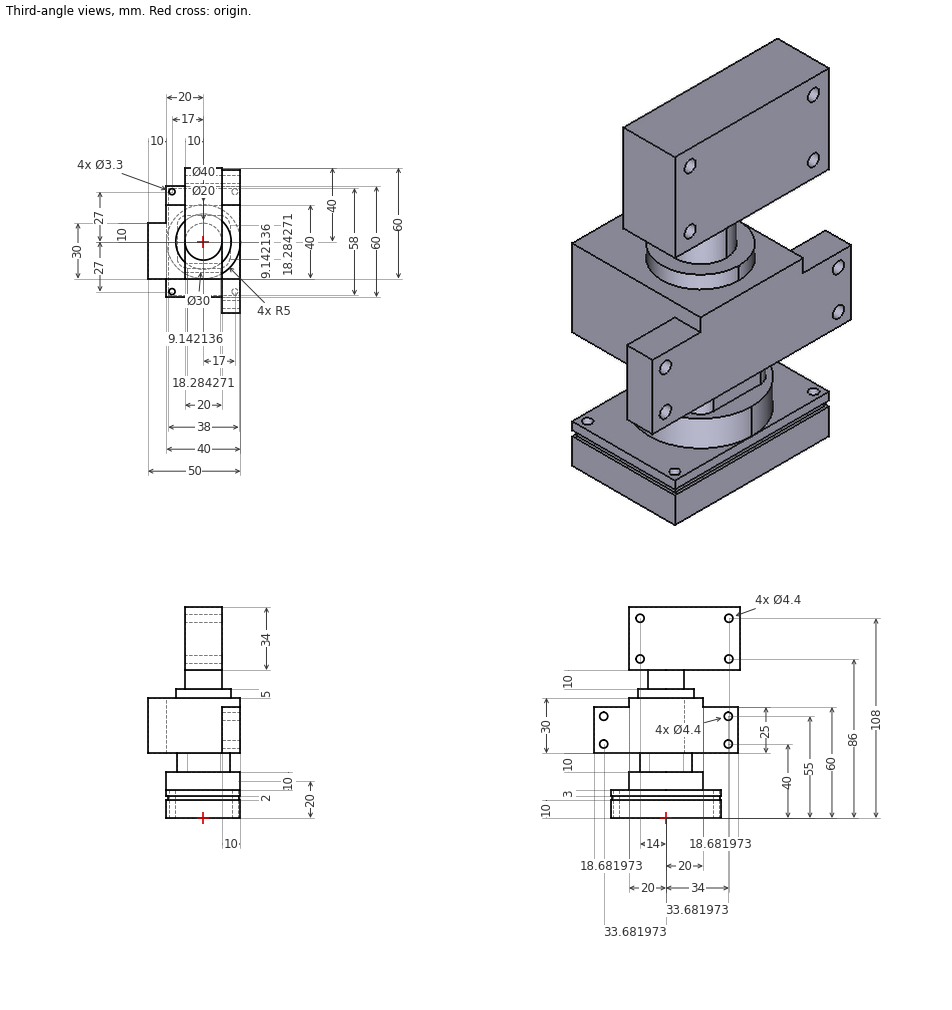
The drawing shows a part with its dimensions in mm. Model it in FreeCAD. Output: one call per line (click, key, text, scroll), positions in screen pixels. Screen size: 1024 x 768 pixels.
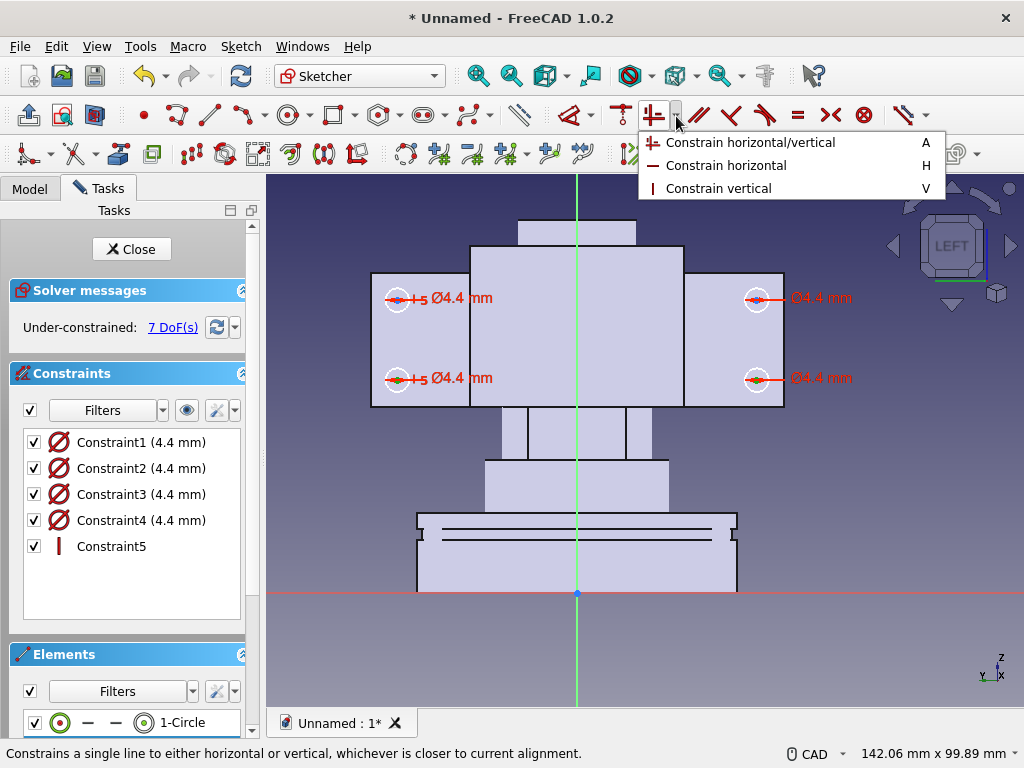
click(792, 166)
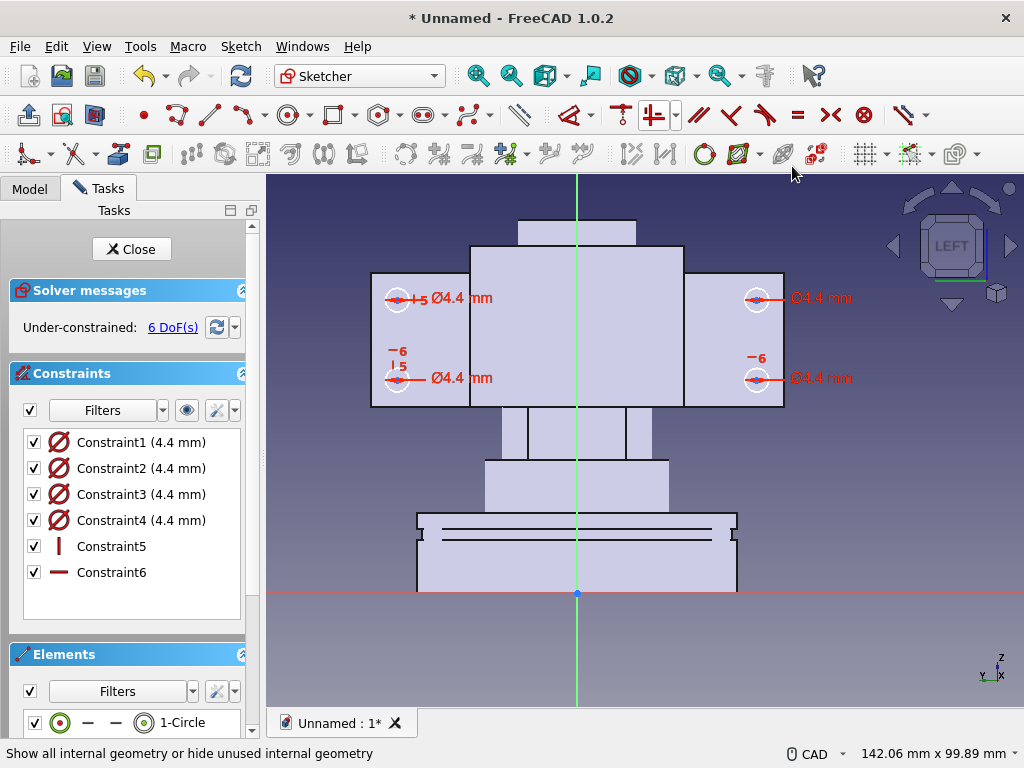
click(757, 380)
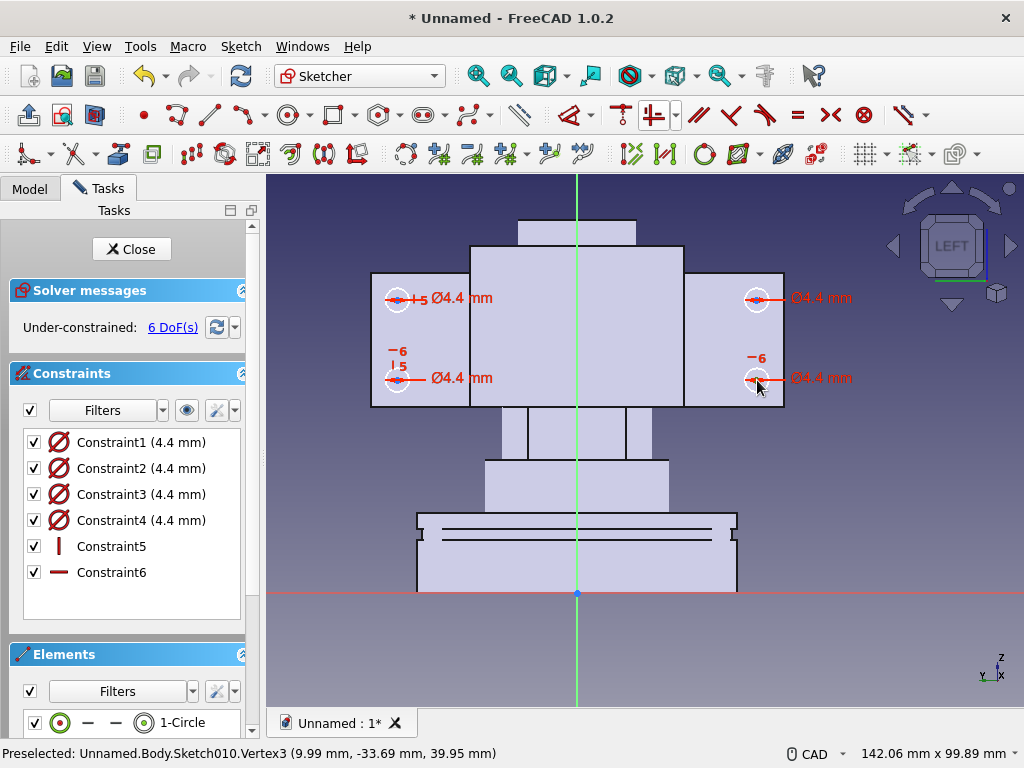
click(757, 300)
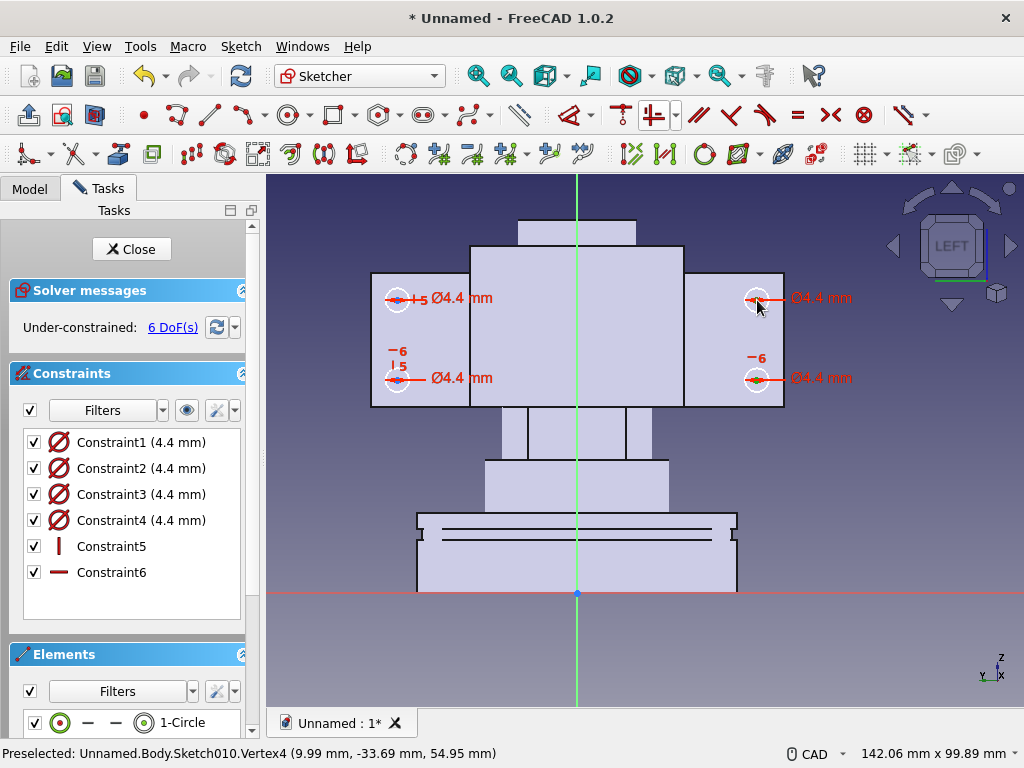
key(v)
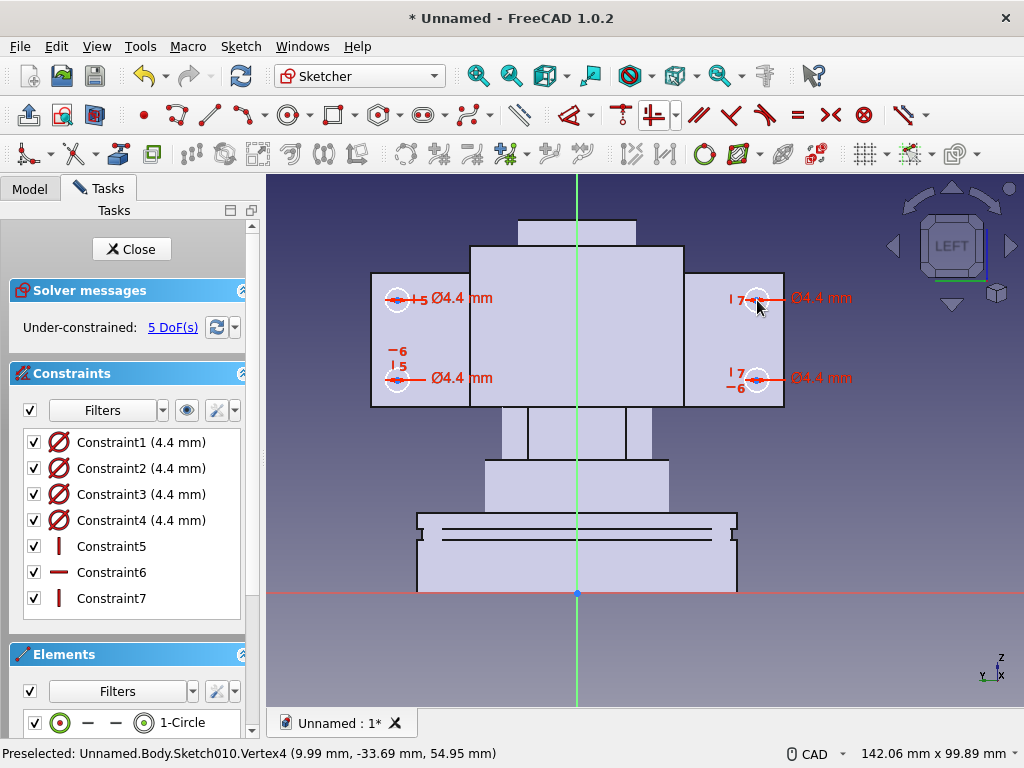
click(397, 300)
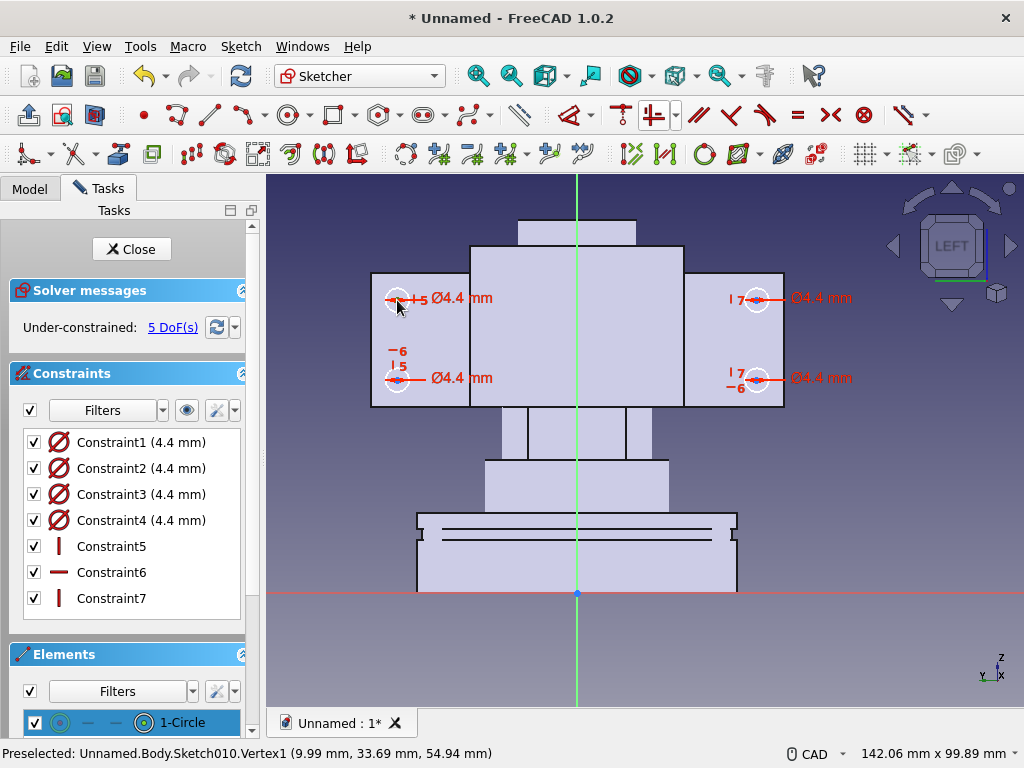
click(757, 300)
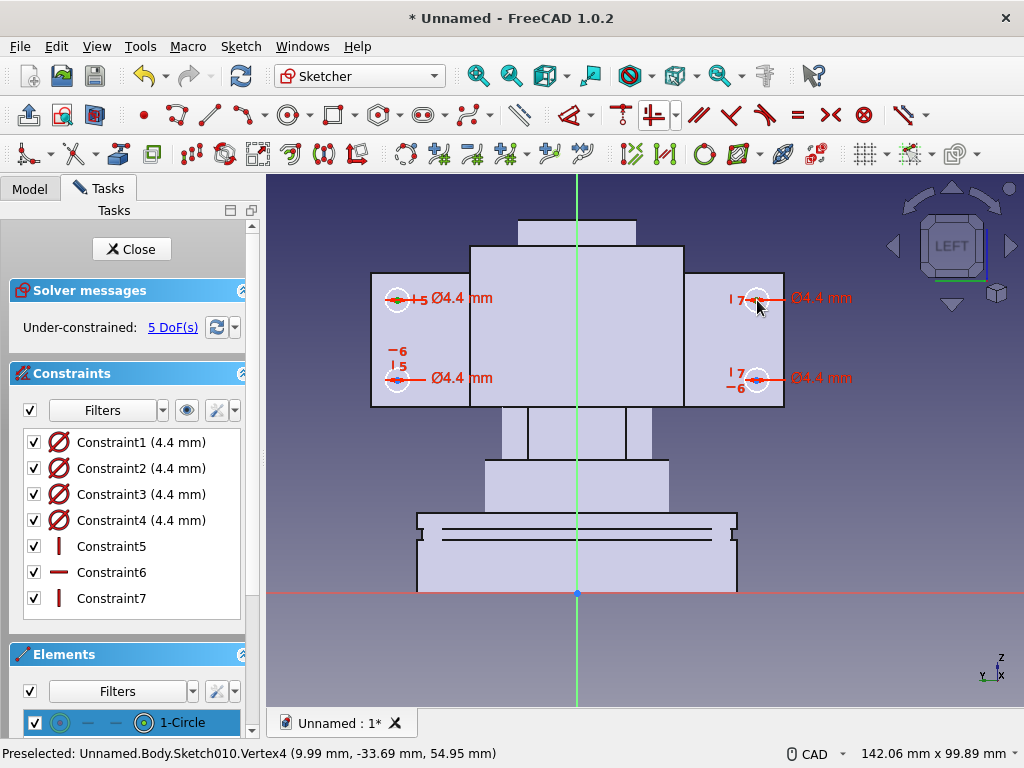
key(h)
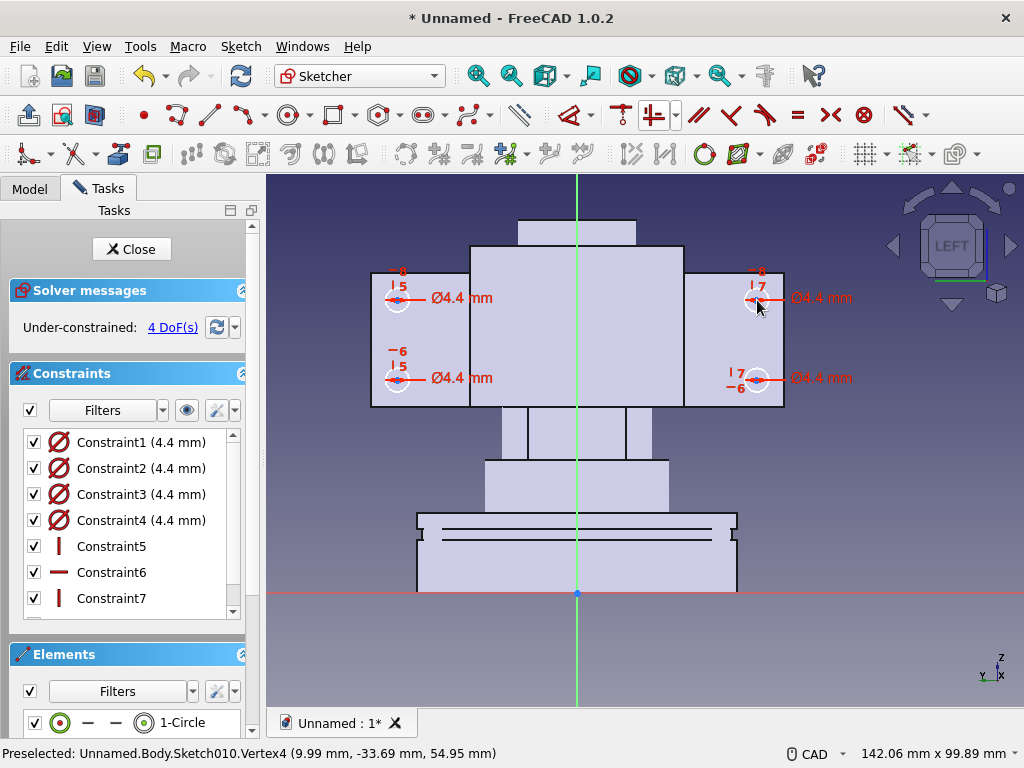
key(d)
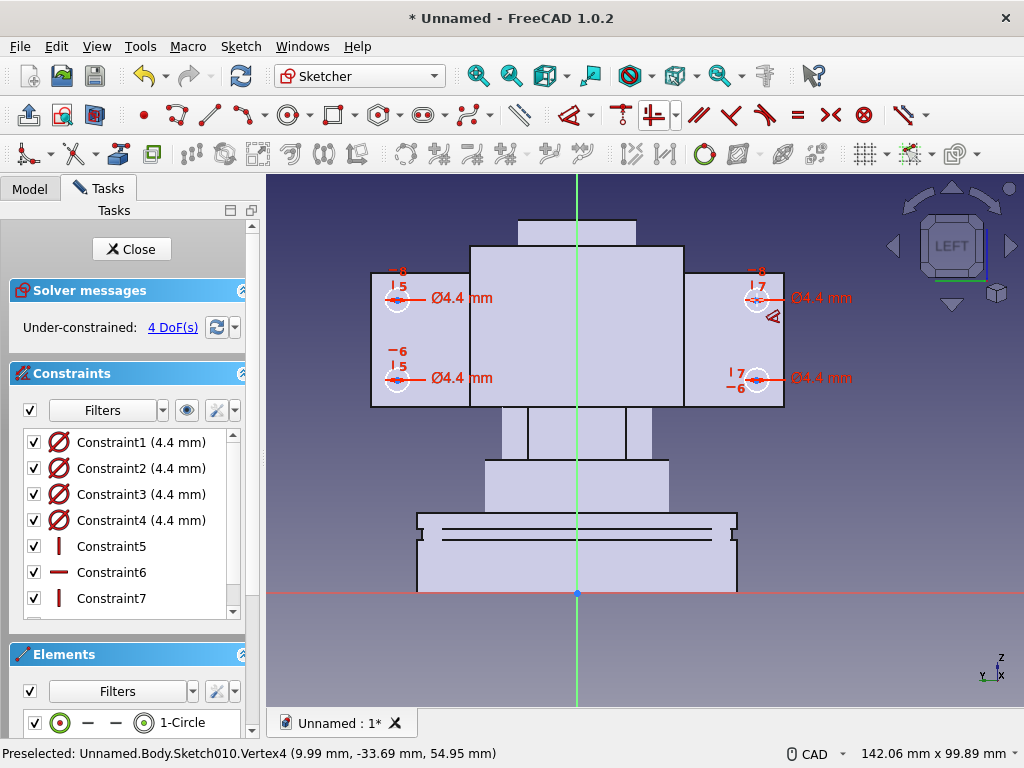
click(397, 300)
click(363, 447)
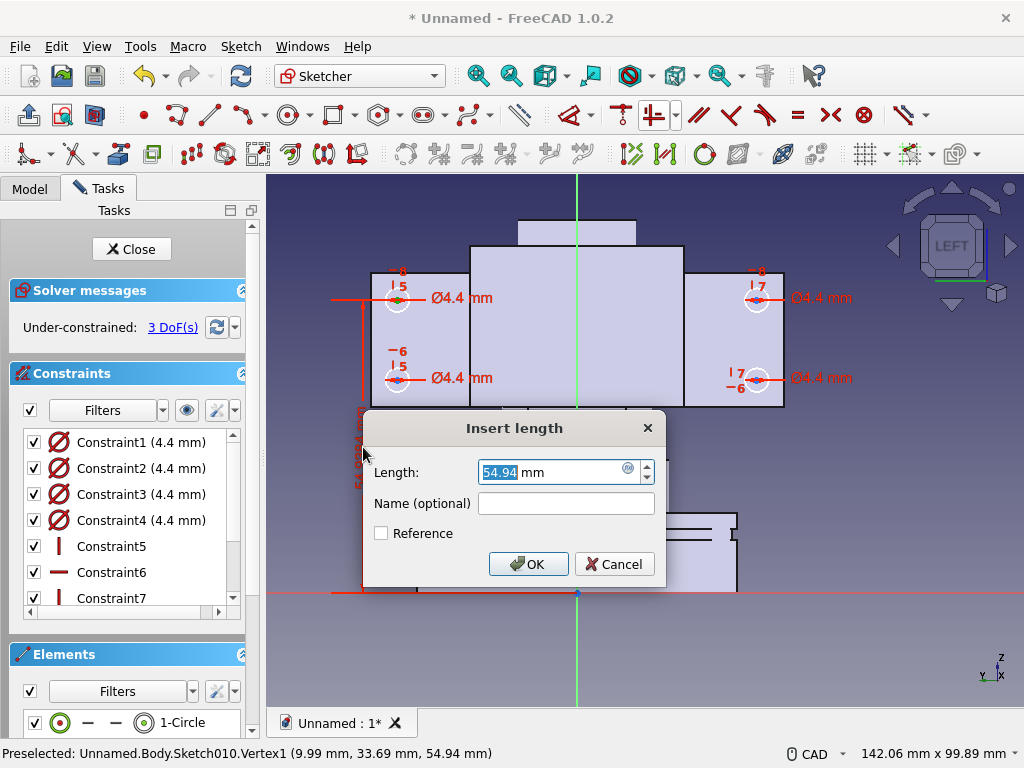
text(55)
key(Return)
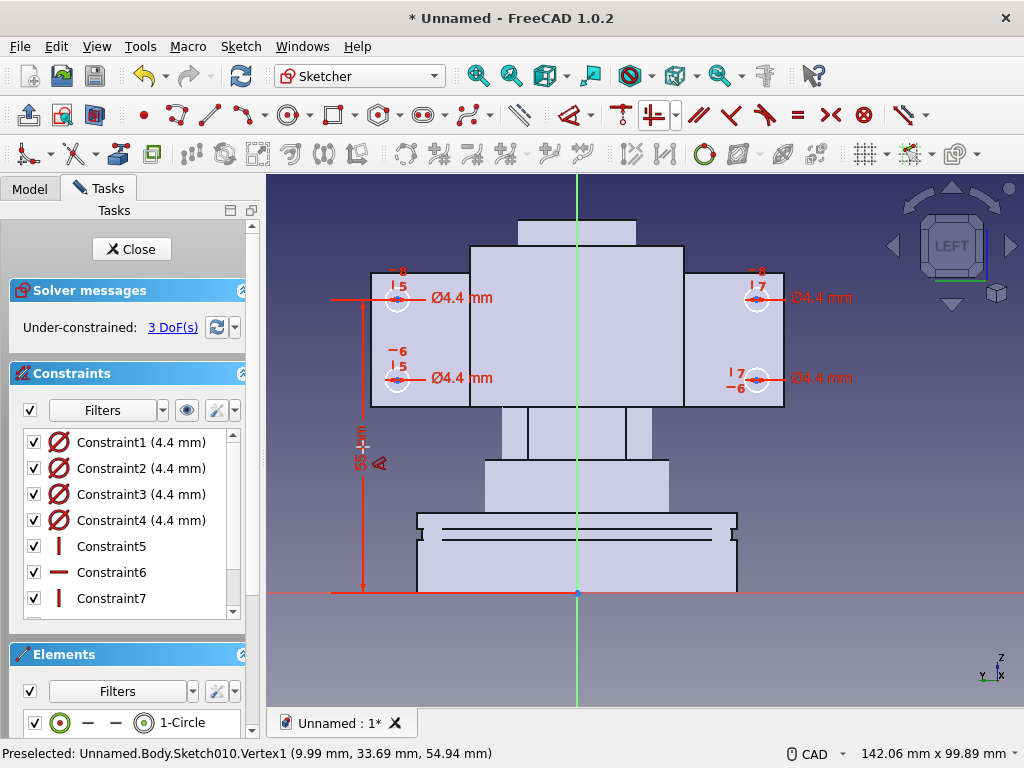
click(397, 380)
click(363, 487)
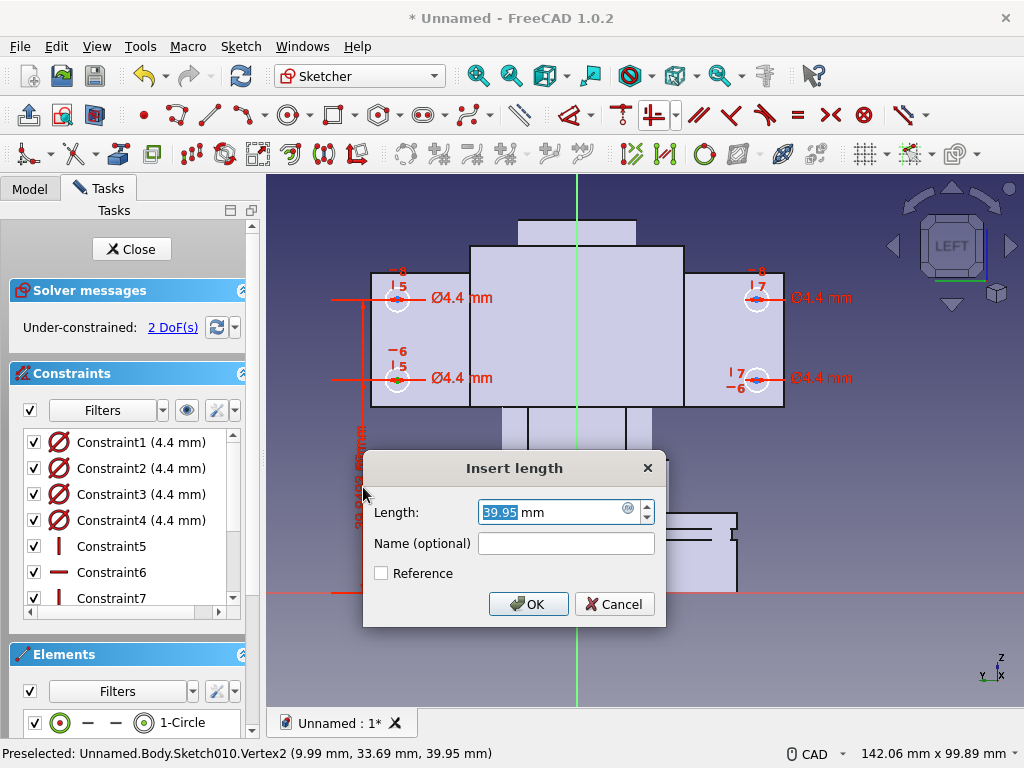
text(40)
key(Return)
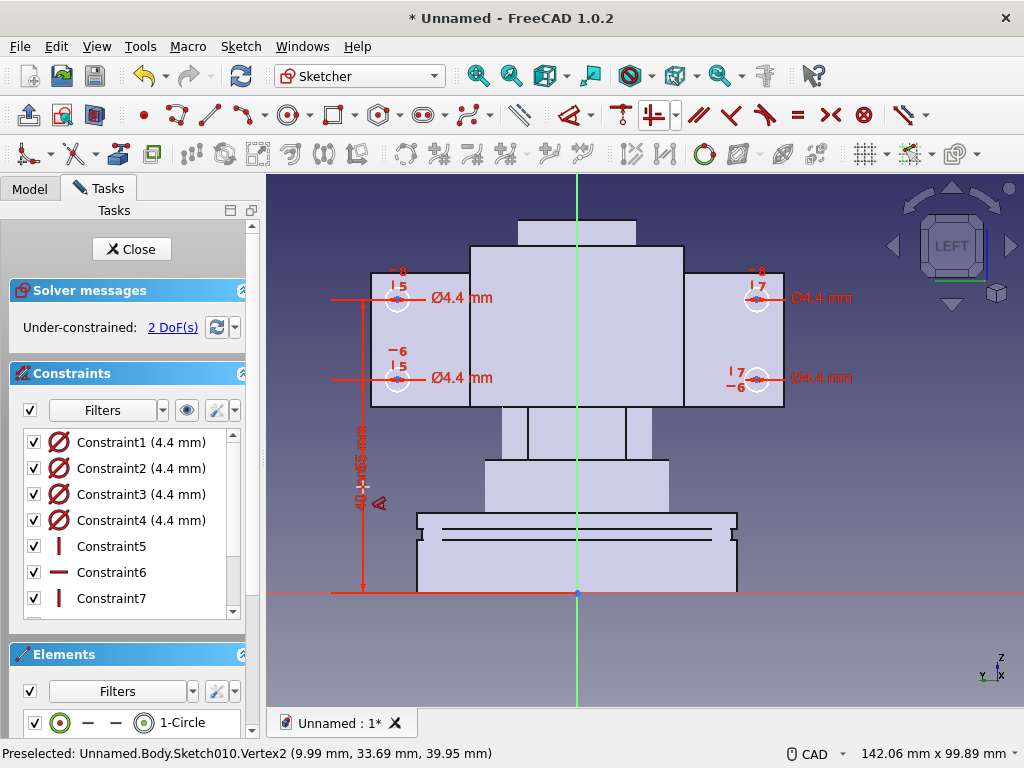
click(397, 300)
click(487, 627)